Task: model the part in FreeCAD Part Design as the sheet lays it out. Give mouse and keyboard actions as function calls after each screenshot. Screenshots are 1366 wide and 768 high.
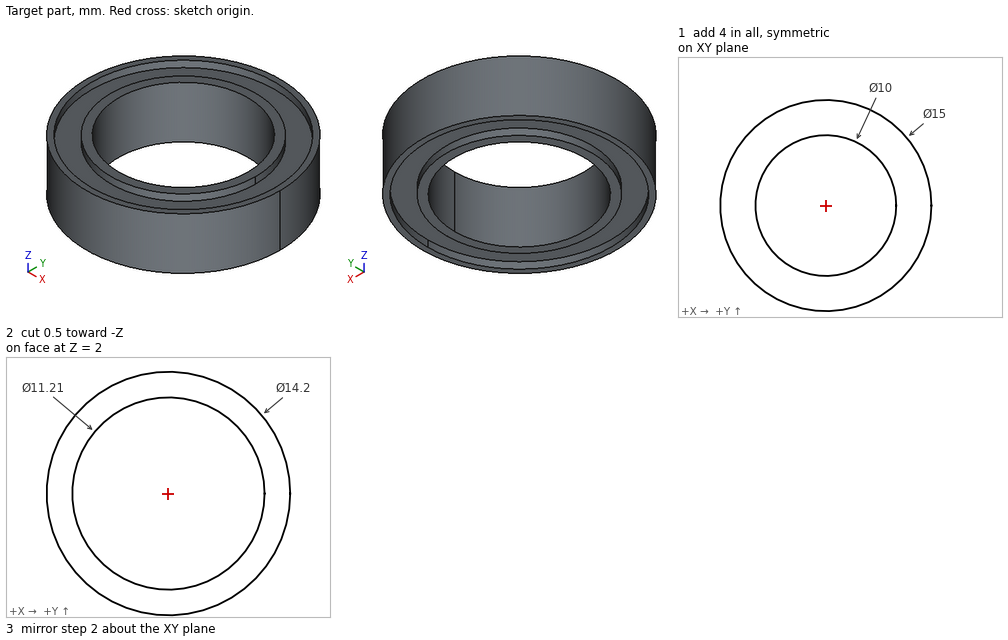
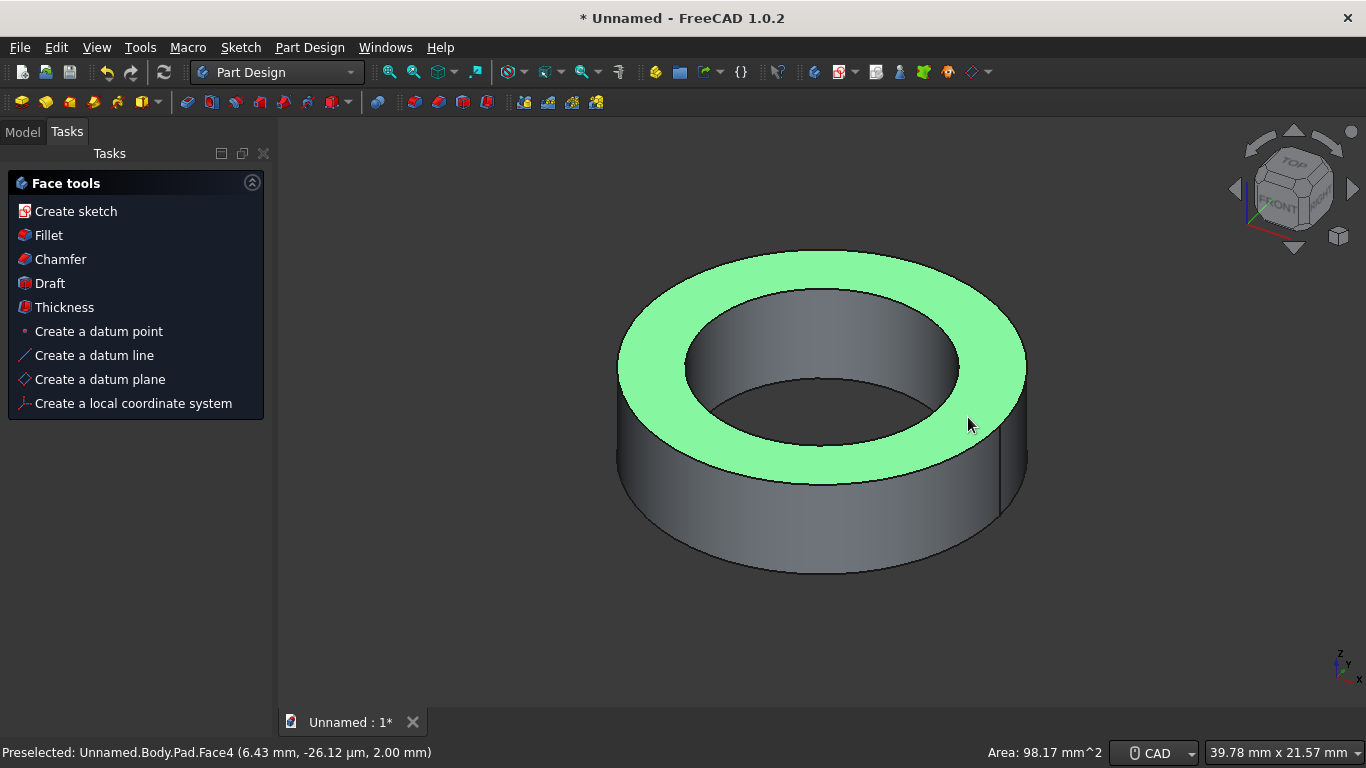
click(840, 72)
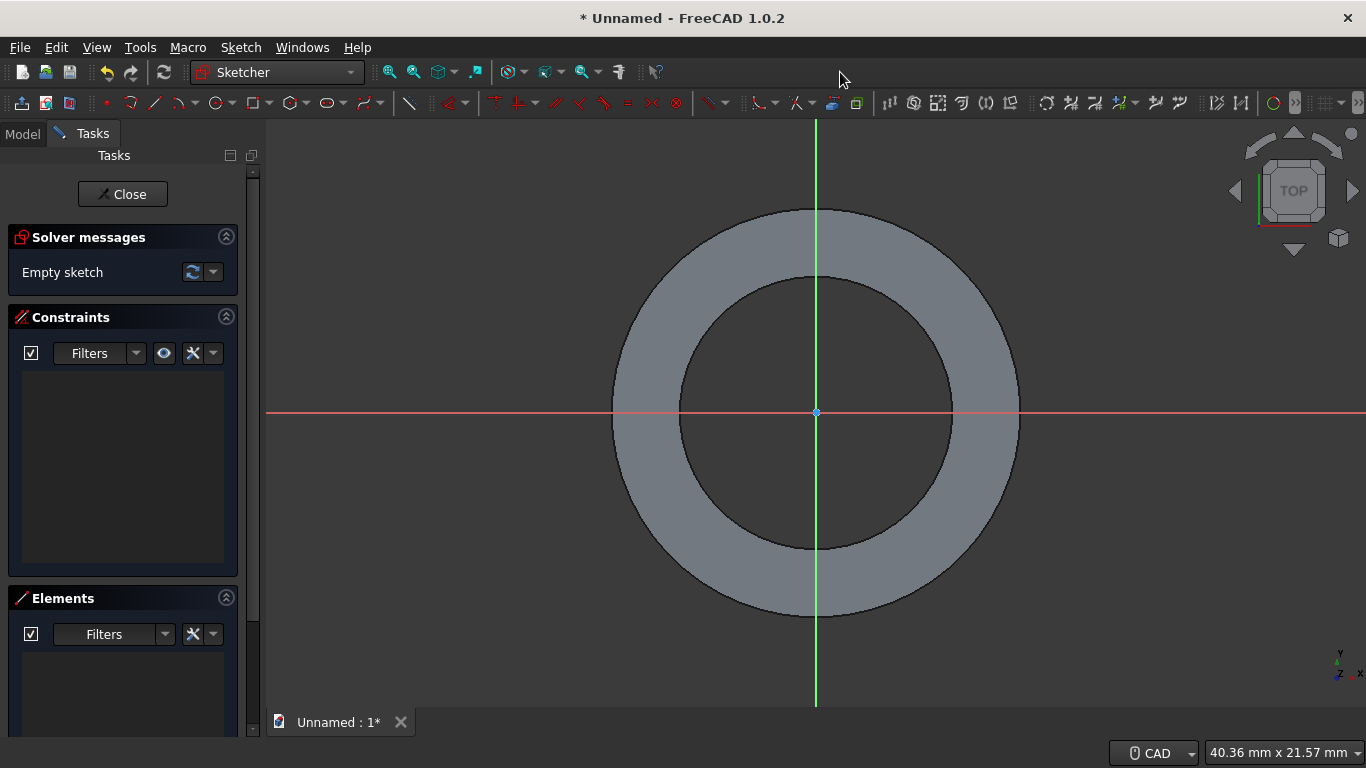
click(216, 104)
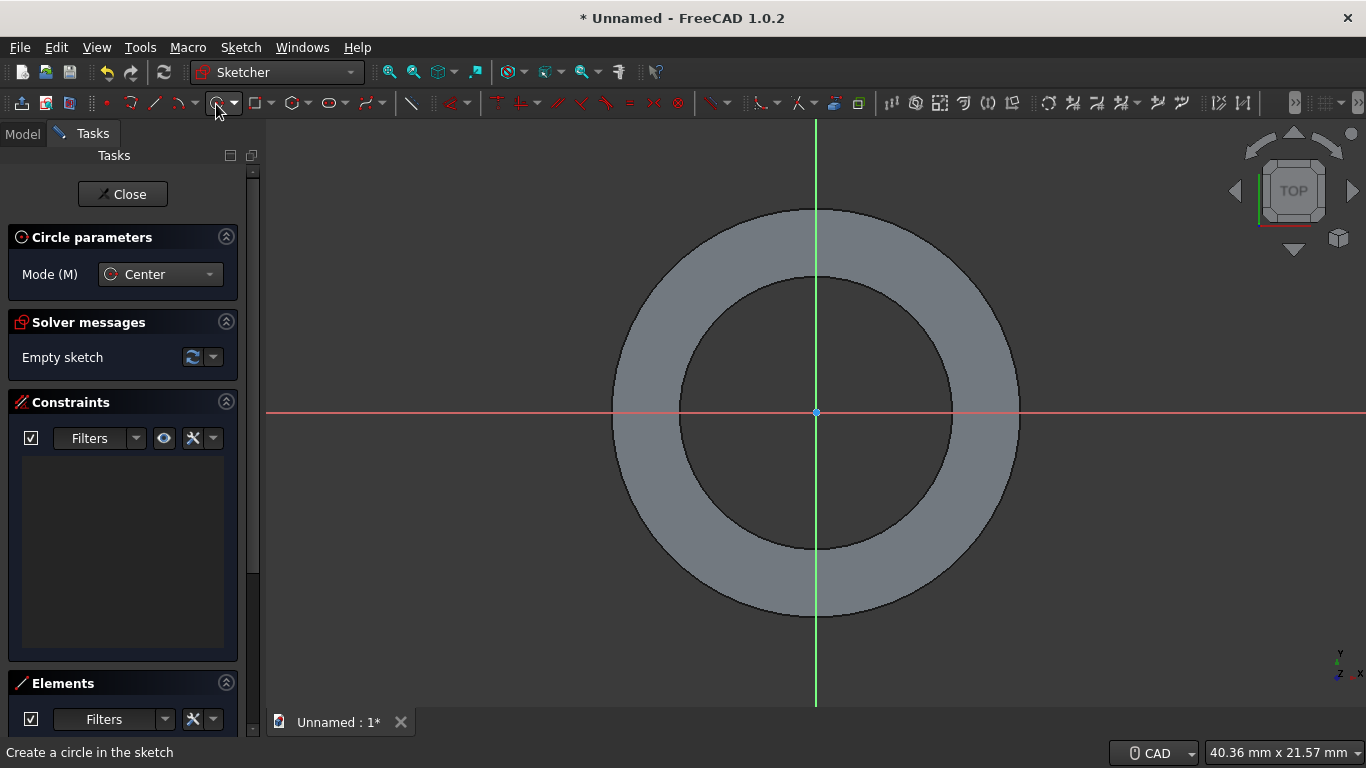
click(816, 413)
click(953, 276)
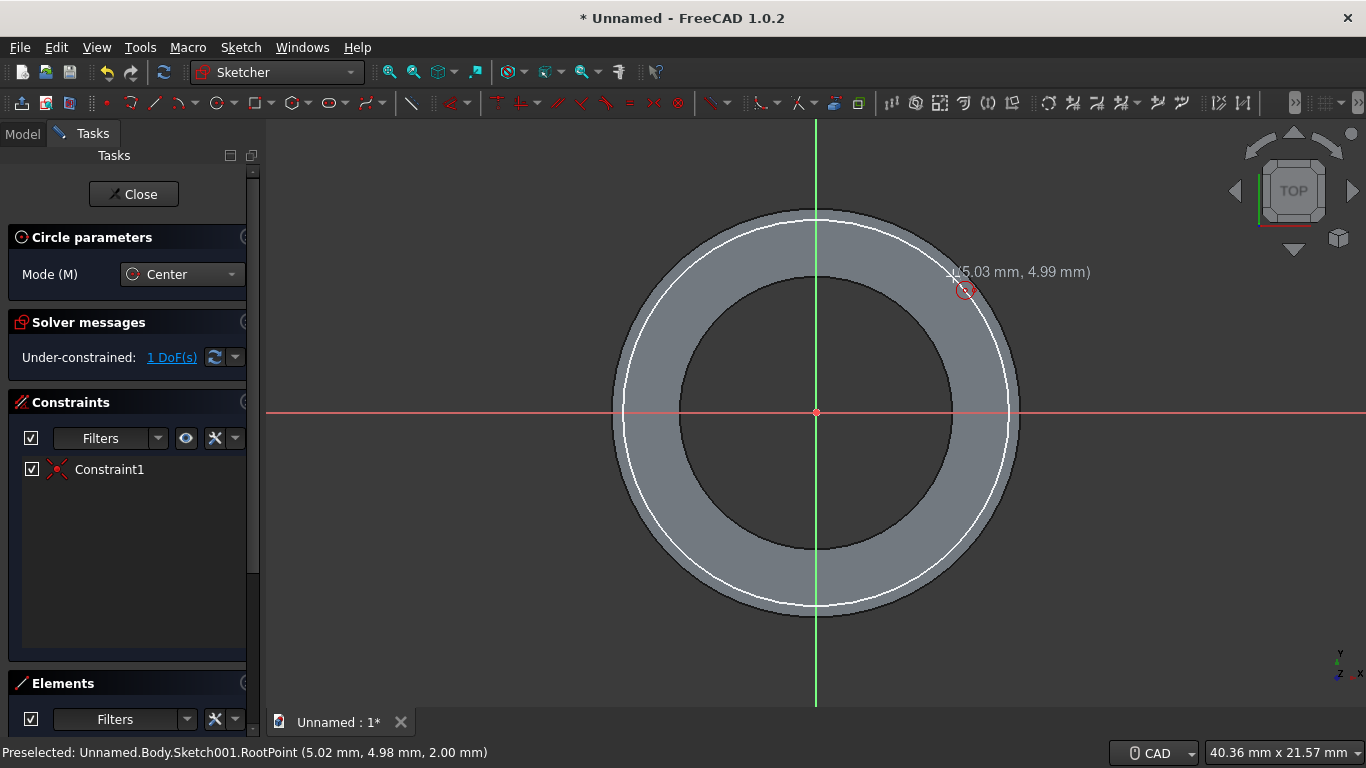
click(816, 413)
click(924, 305)
key(Escape)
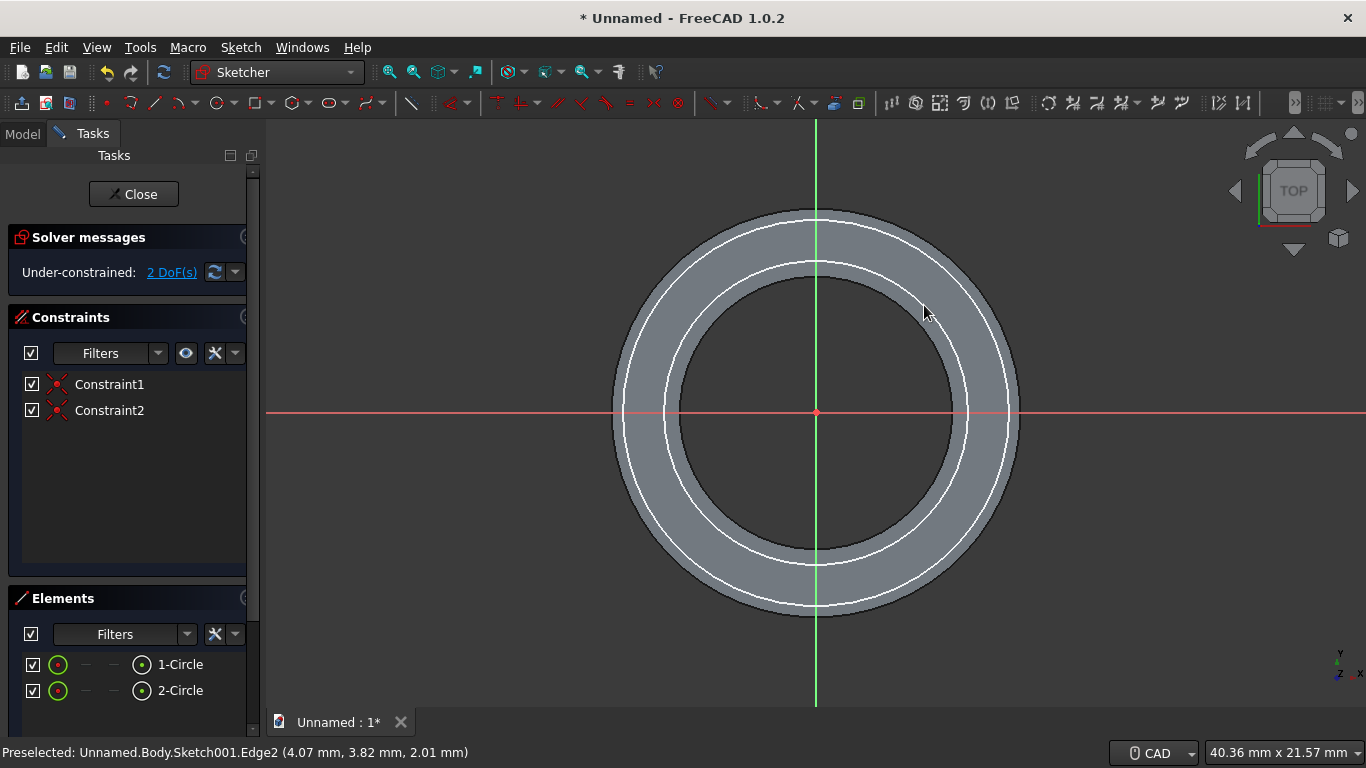
click(450, 104)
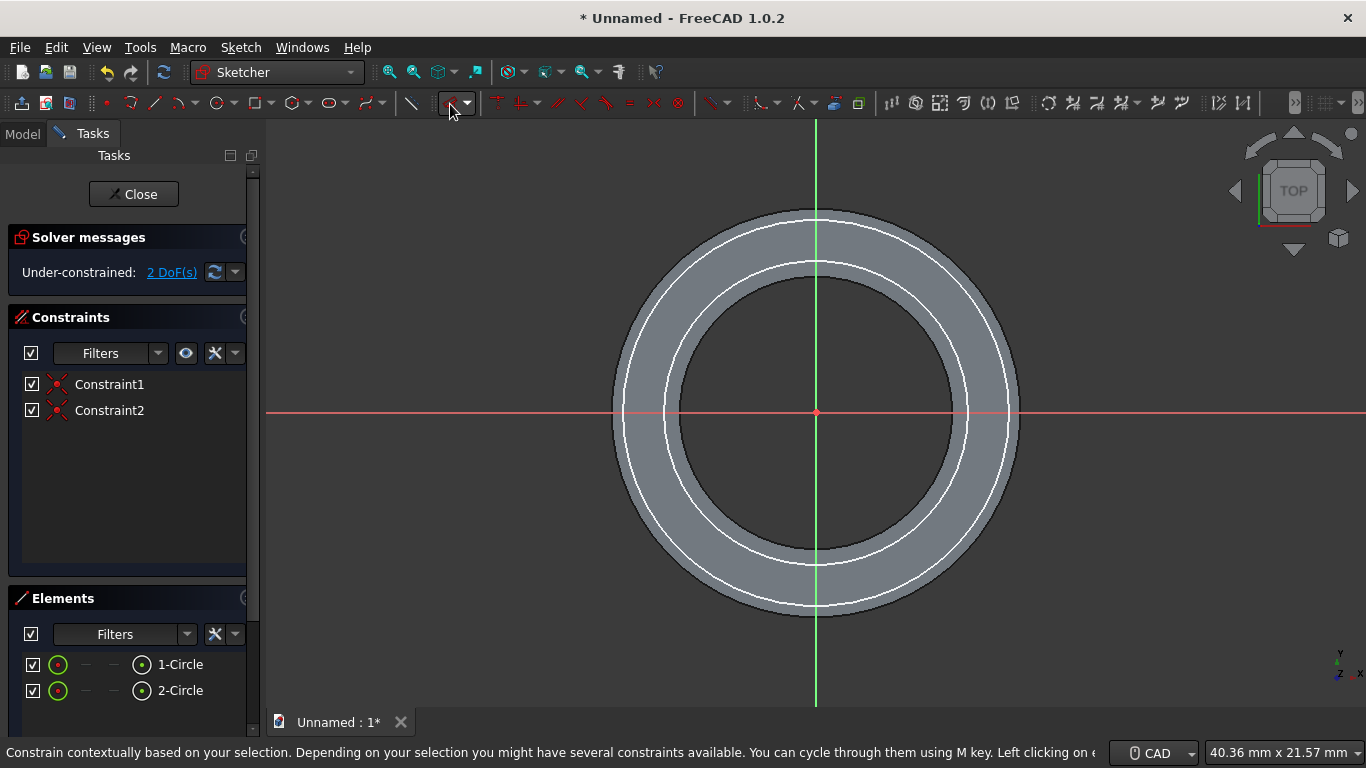
click(952, 276)
click(975, 253)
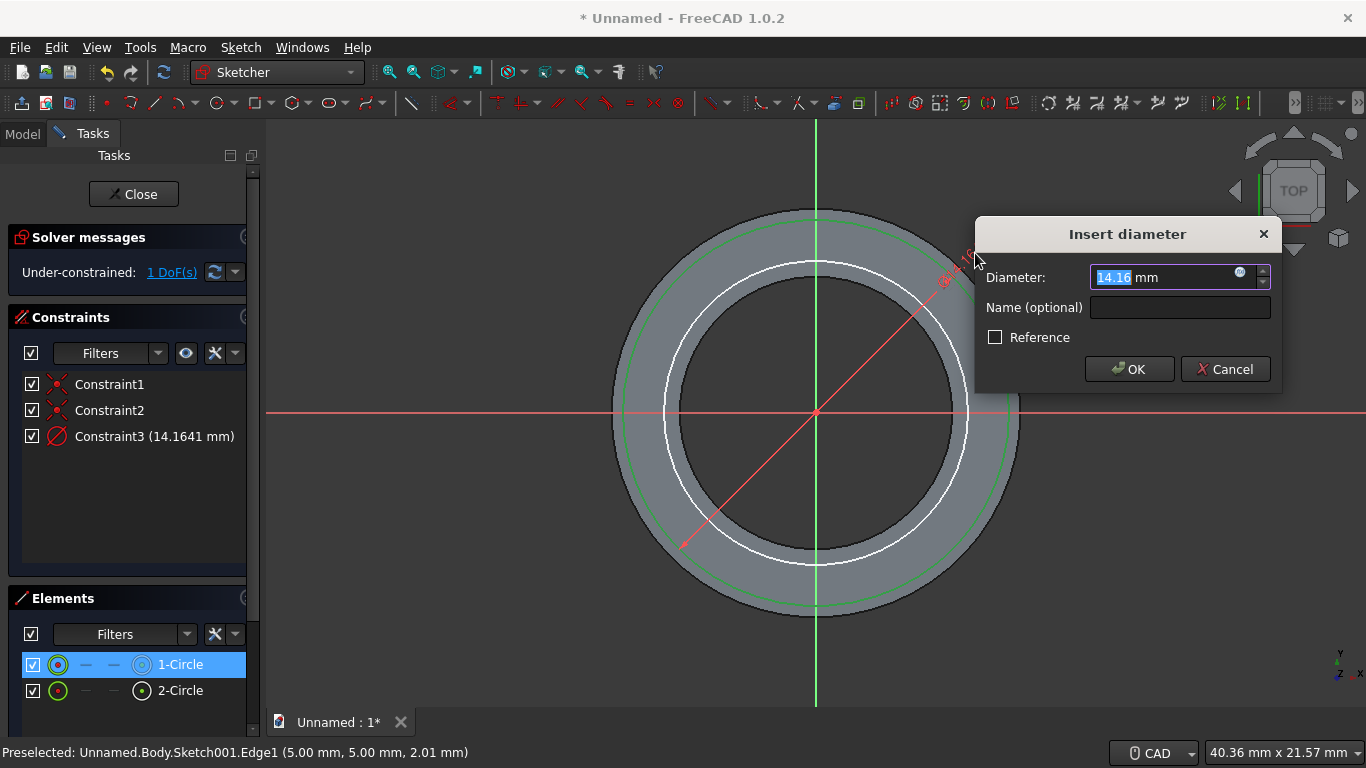
text(14.2)
key(Return)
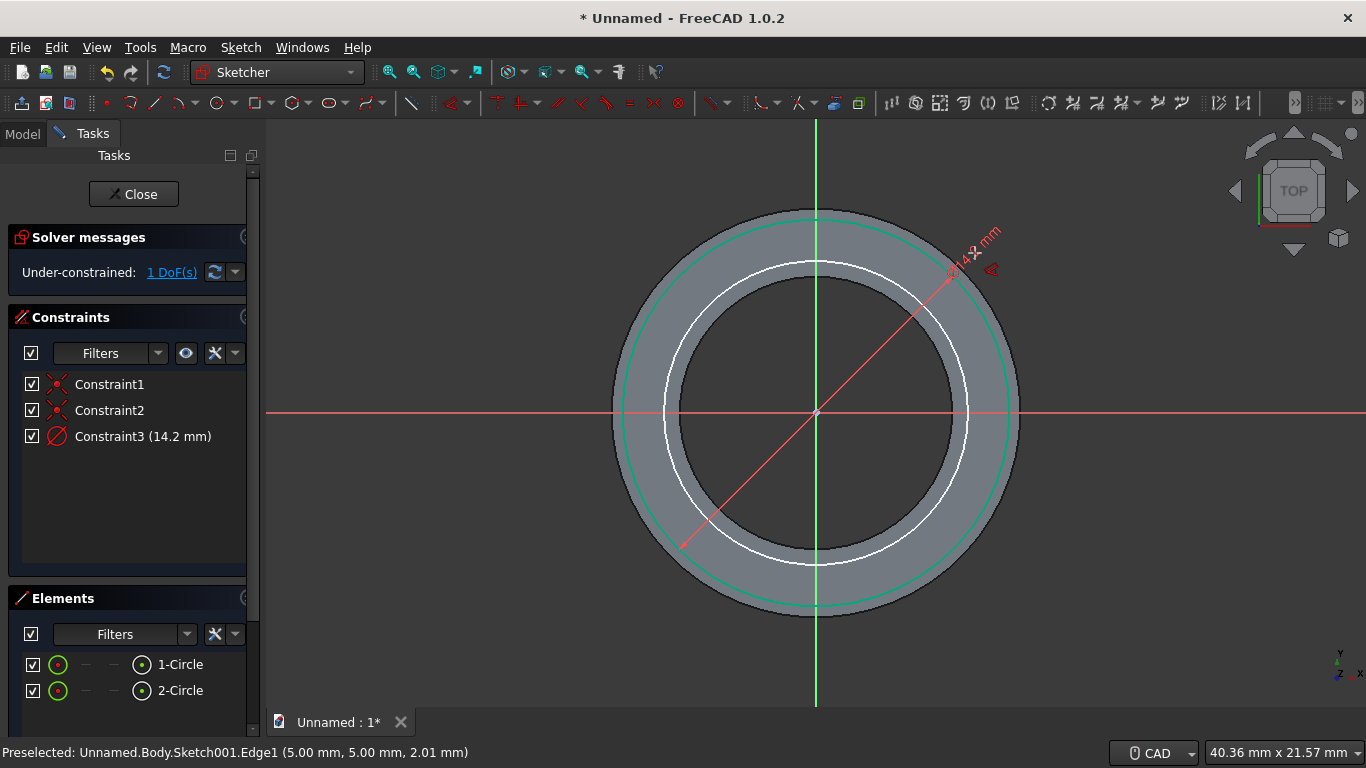
click(923, 305)
click(1014, 354)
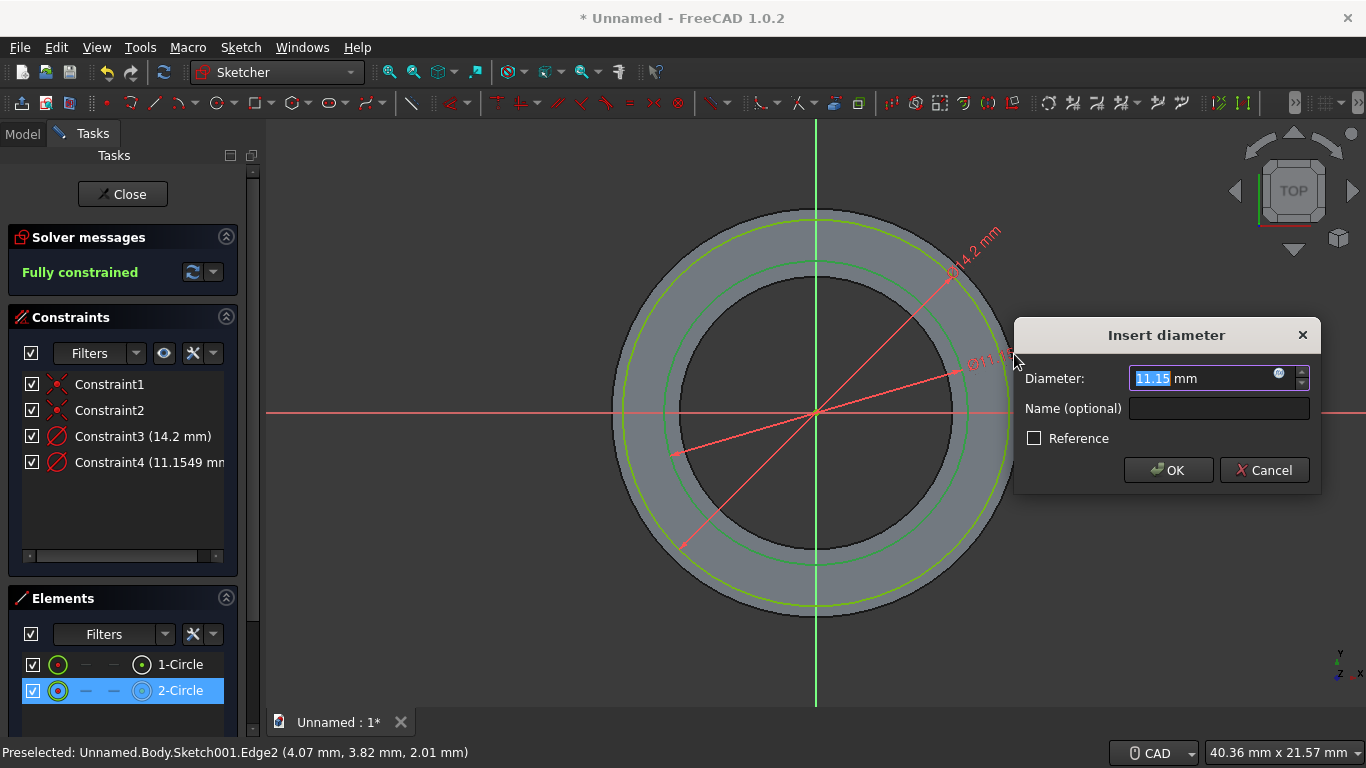
text(11.21)
key(Return)
key(Escape)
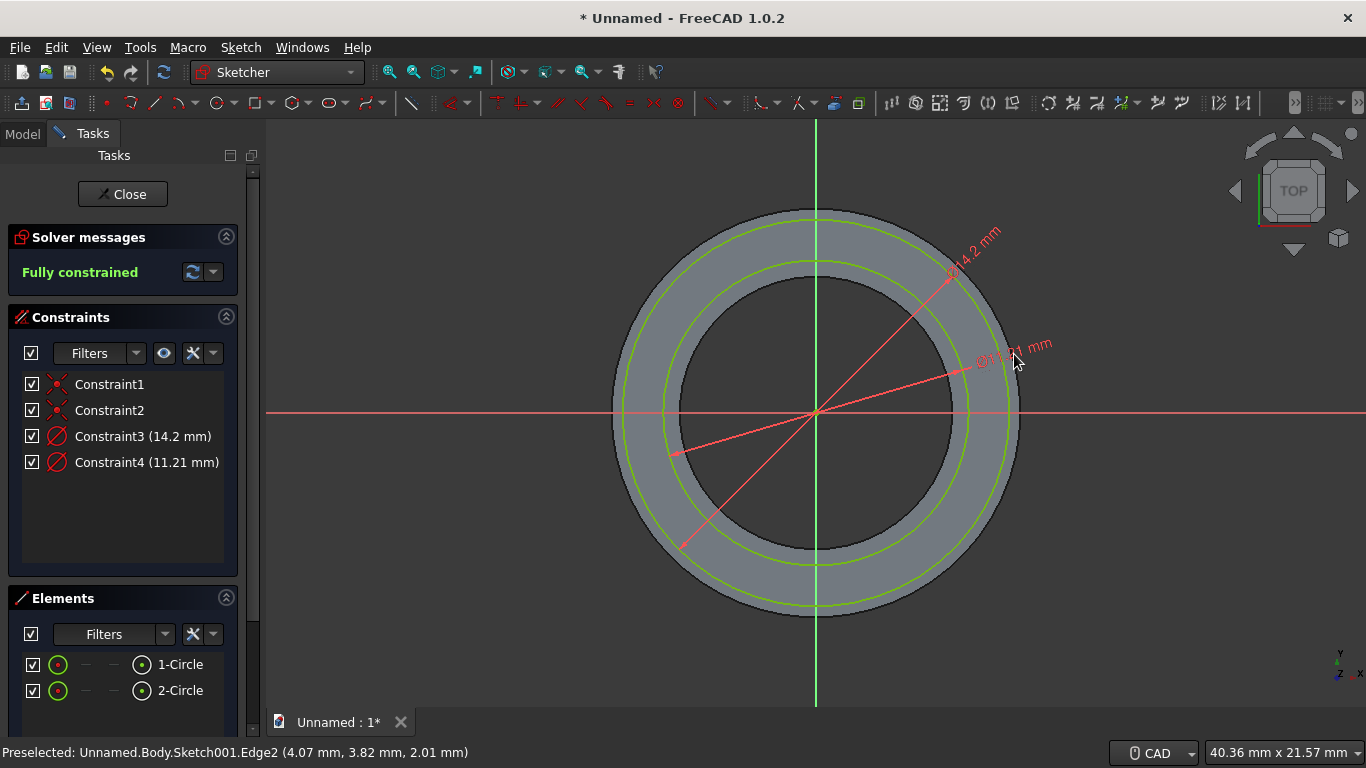
click(123, 194)